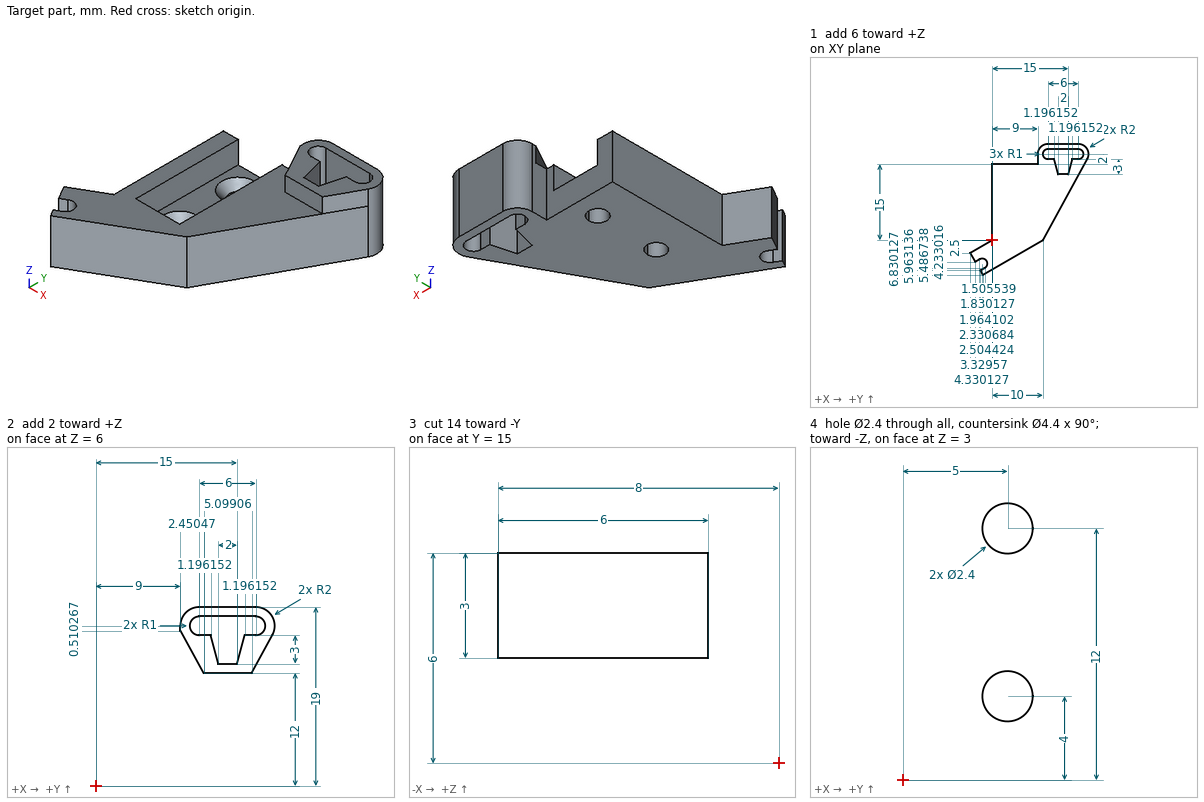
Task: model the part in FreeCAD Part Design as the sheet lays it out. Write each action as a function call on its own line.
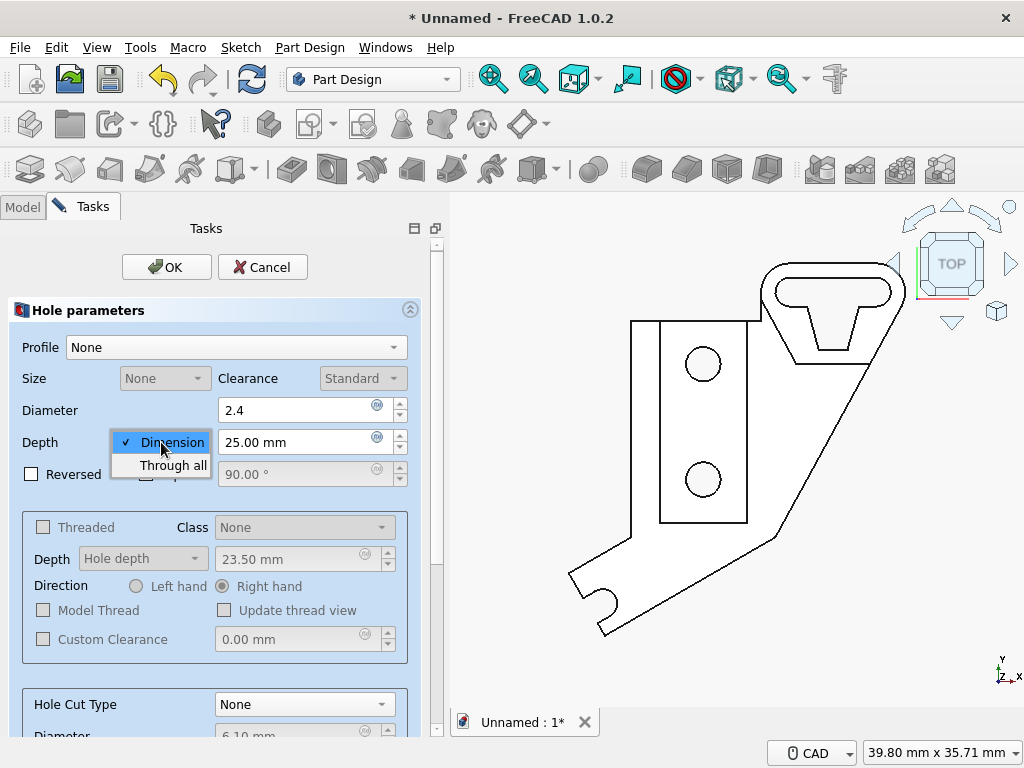
click(160, 466)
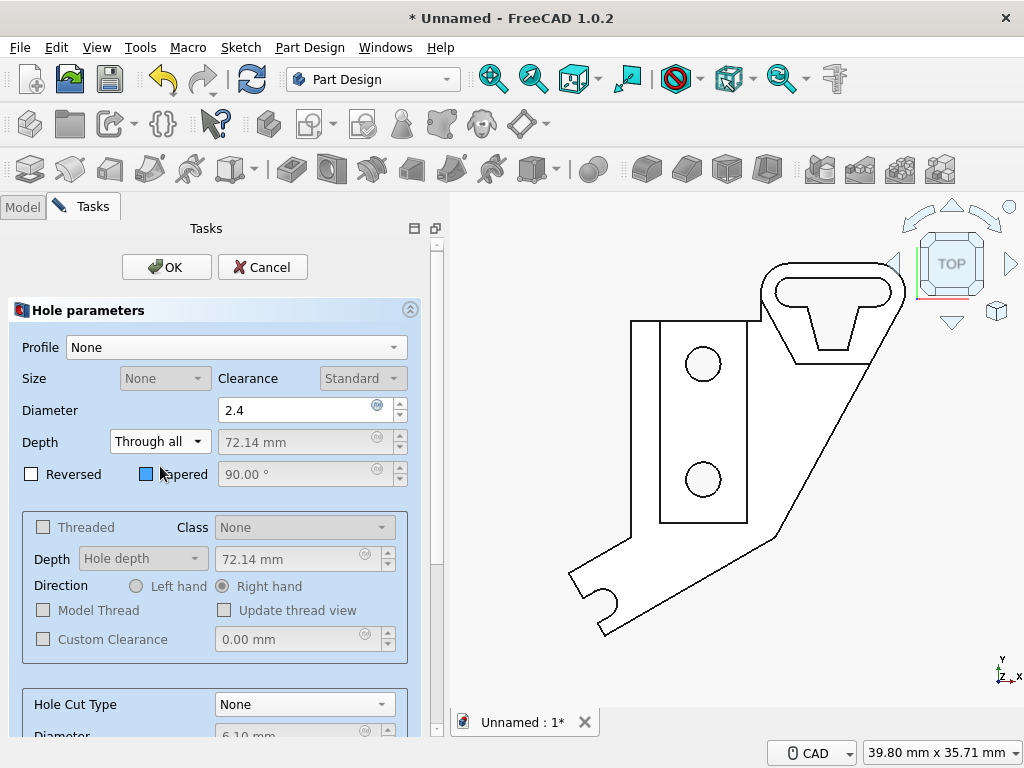
click(306, 704)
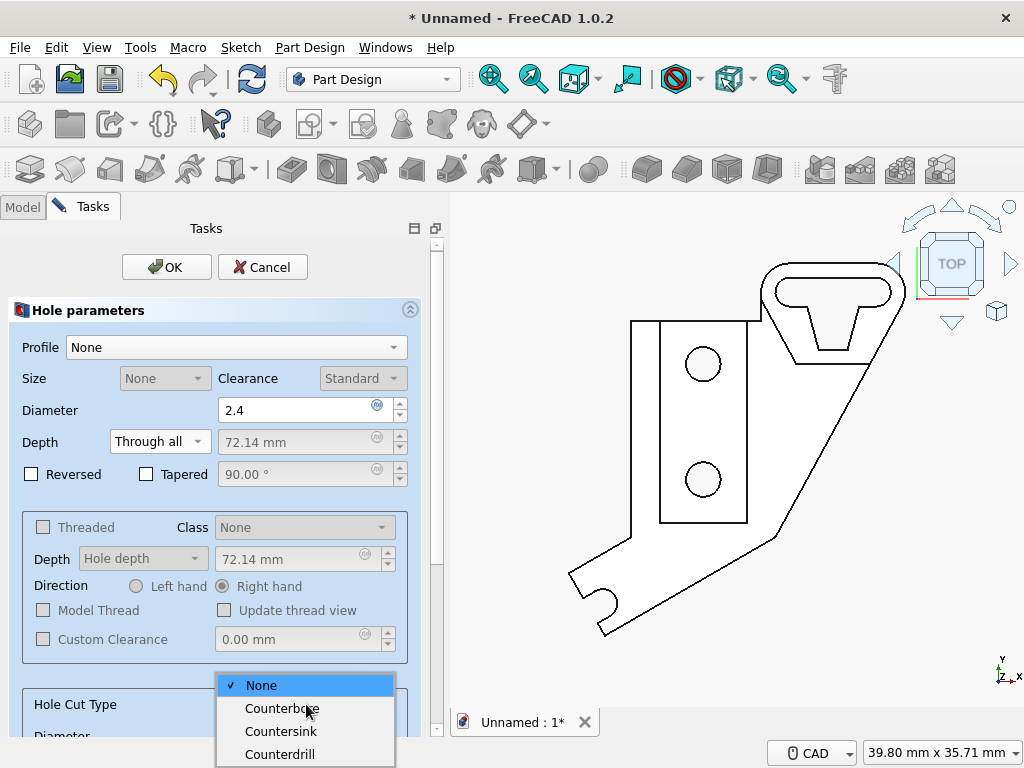
click(304, 732)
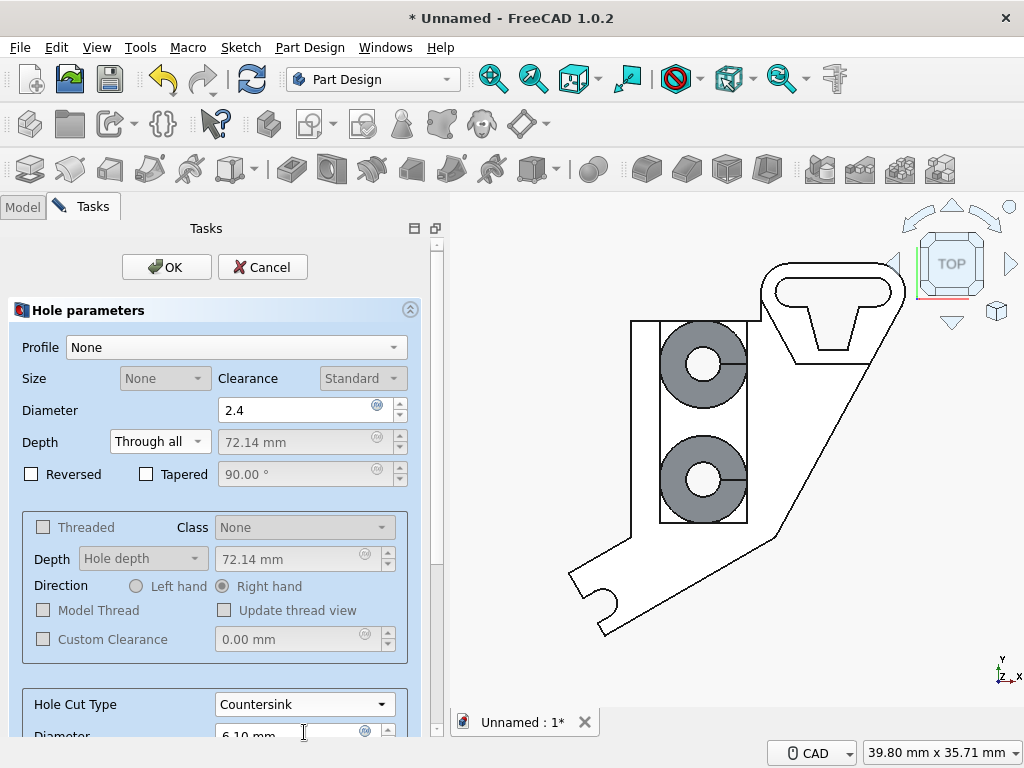
scroll(437, 487, down, 2)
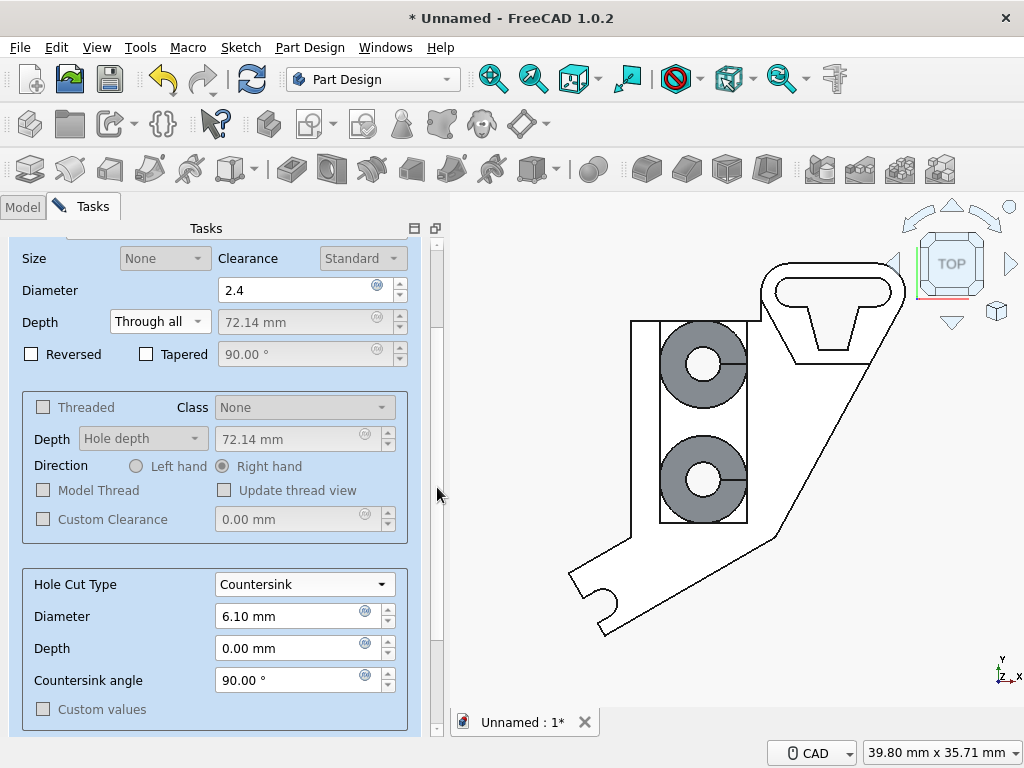
triple_click(298, 616)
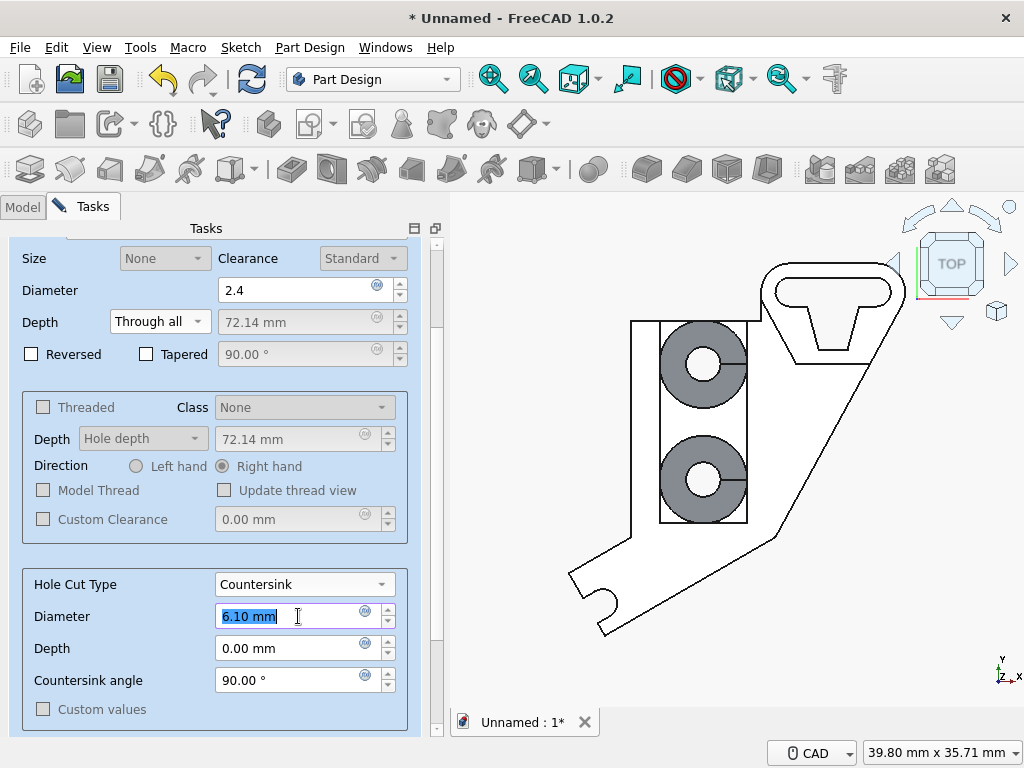
text(4.4)
key(Tab)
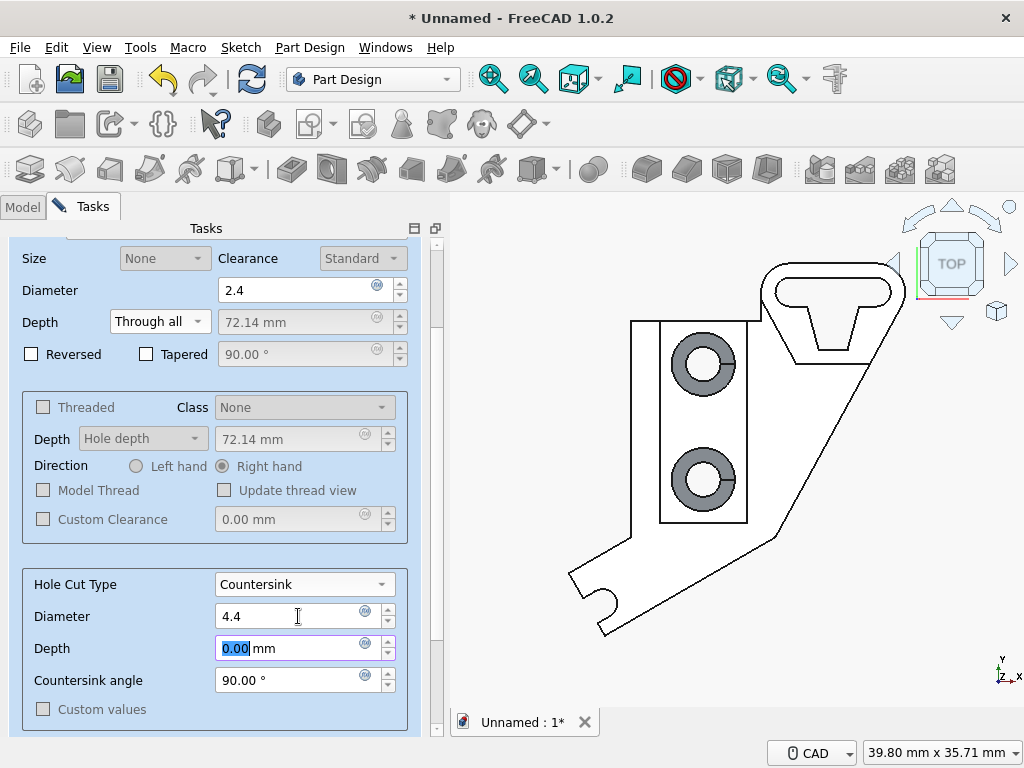
scroll(437, 487, up, 3)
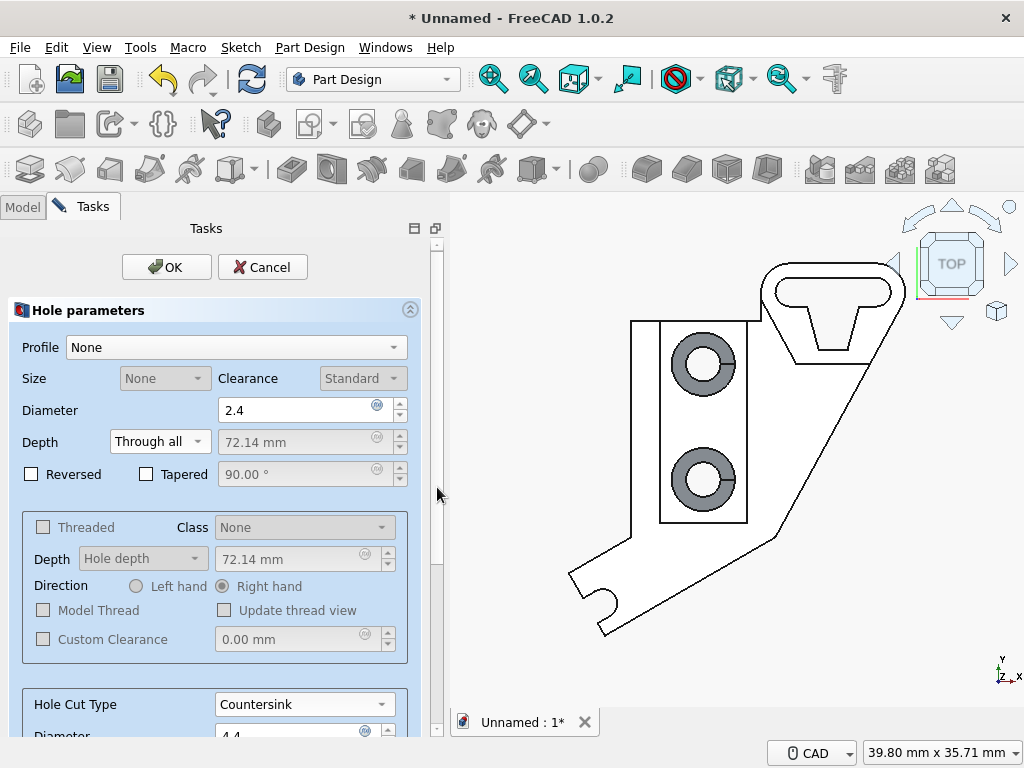
click(167, 267)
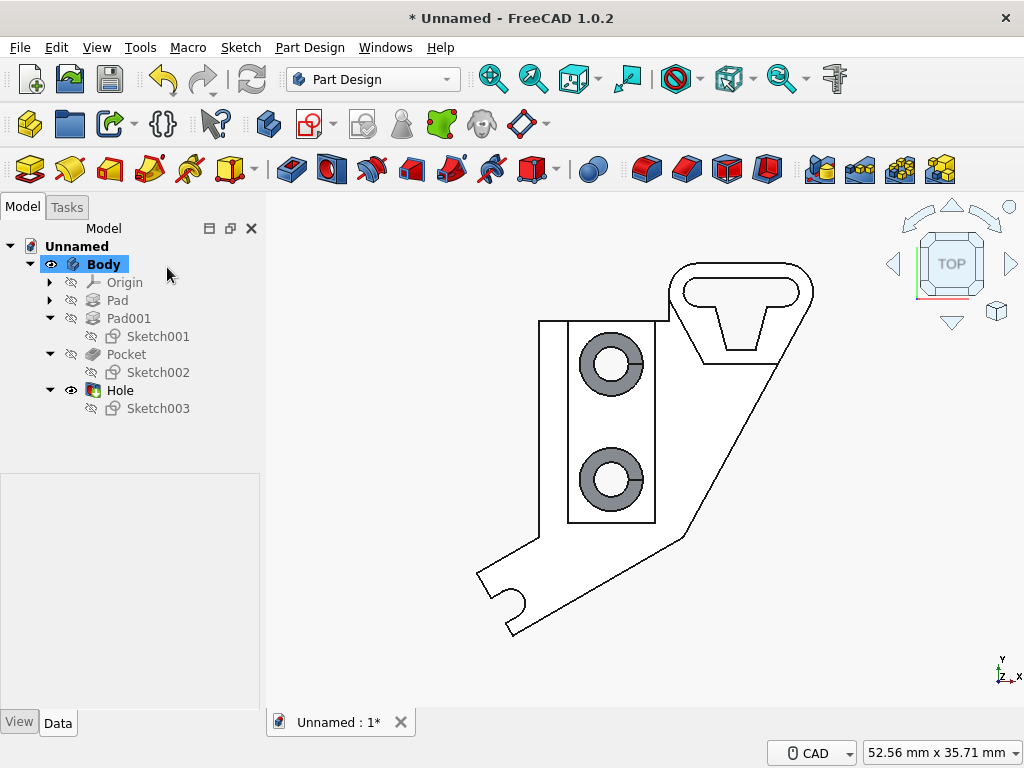
key(0)